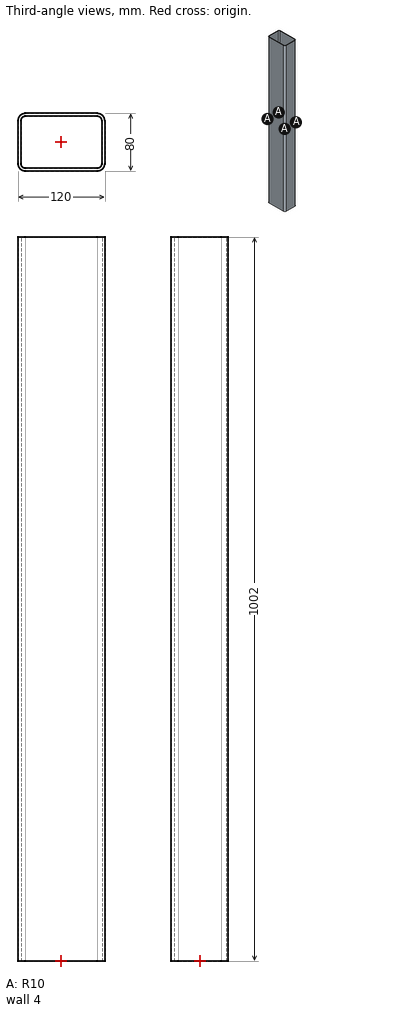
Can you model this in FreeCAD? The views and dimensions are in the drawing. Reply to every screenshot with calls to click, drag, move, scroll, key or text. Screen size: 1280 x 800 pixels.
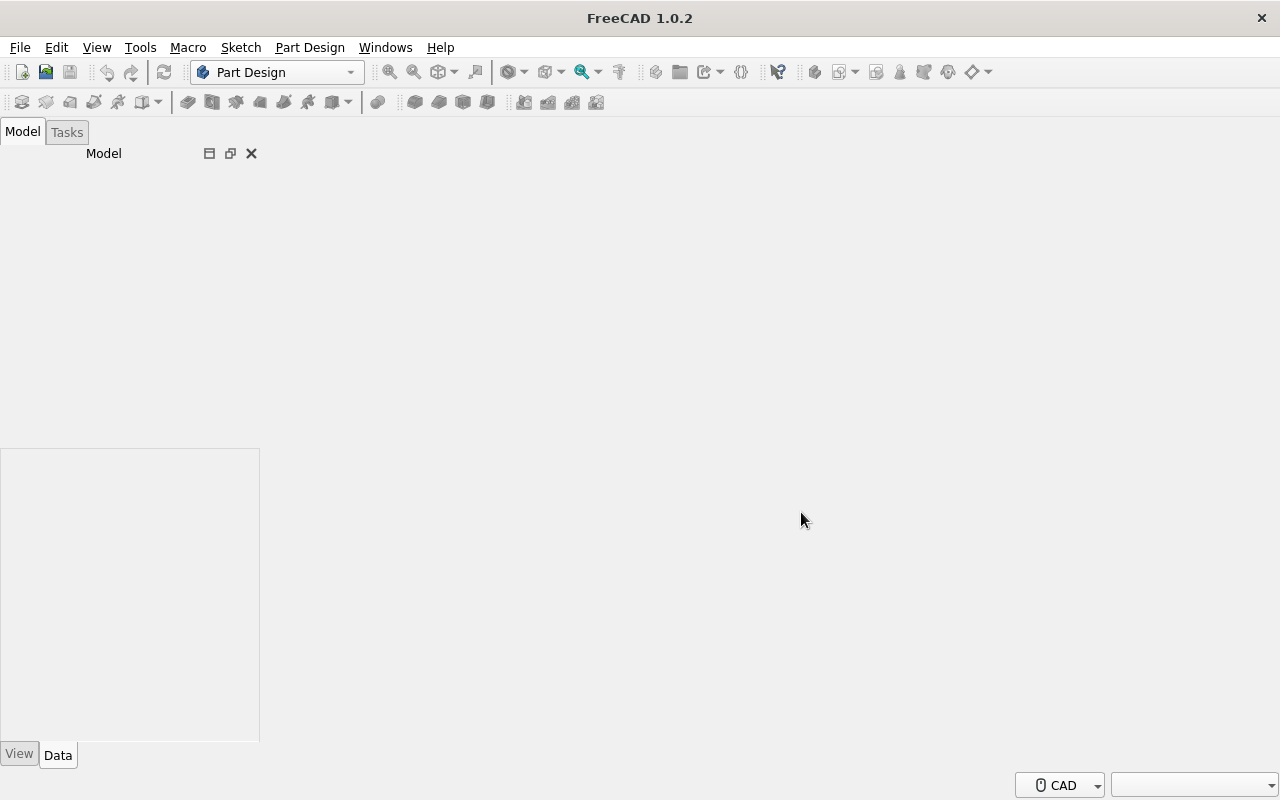
click(22, 72)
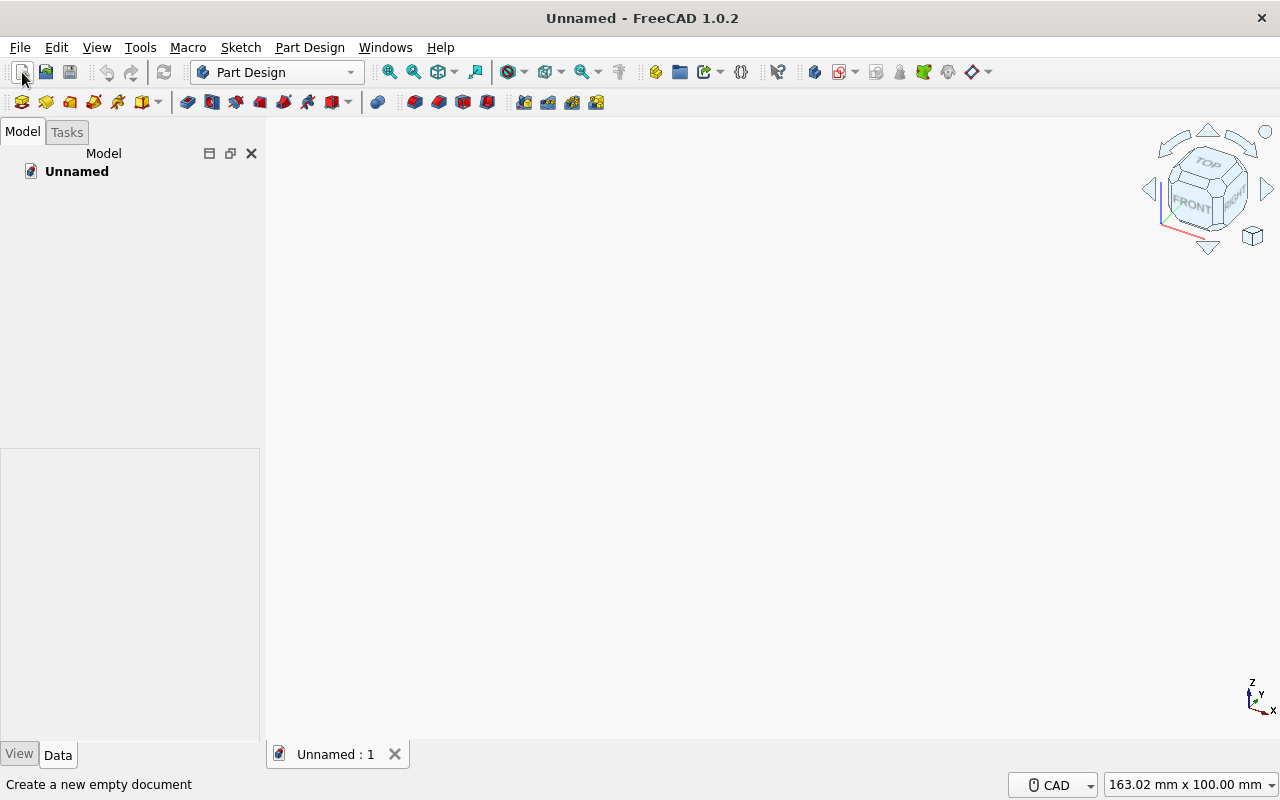
click(840, 72)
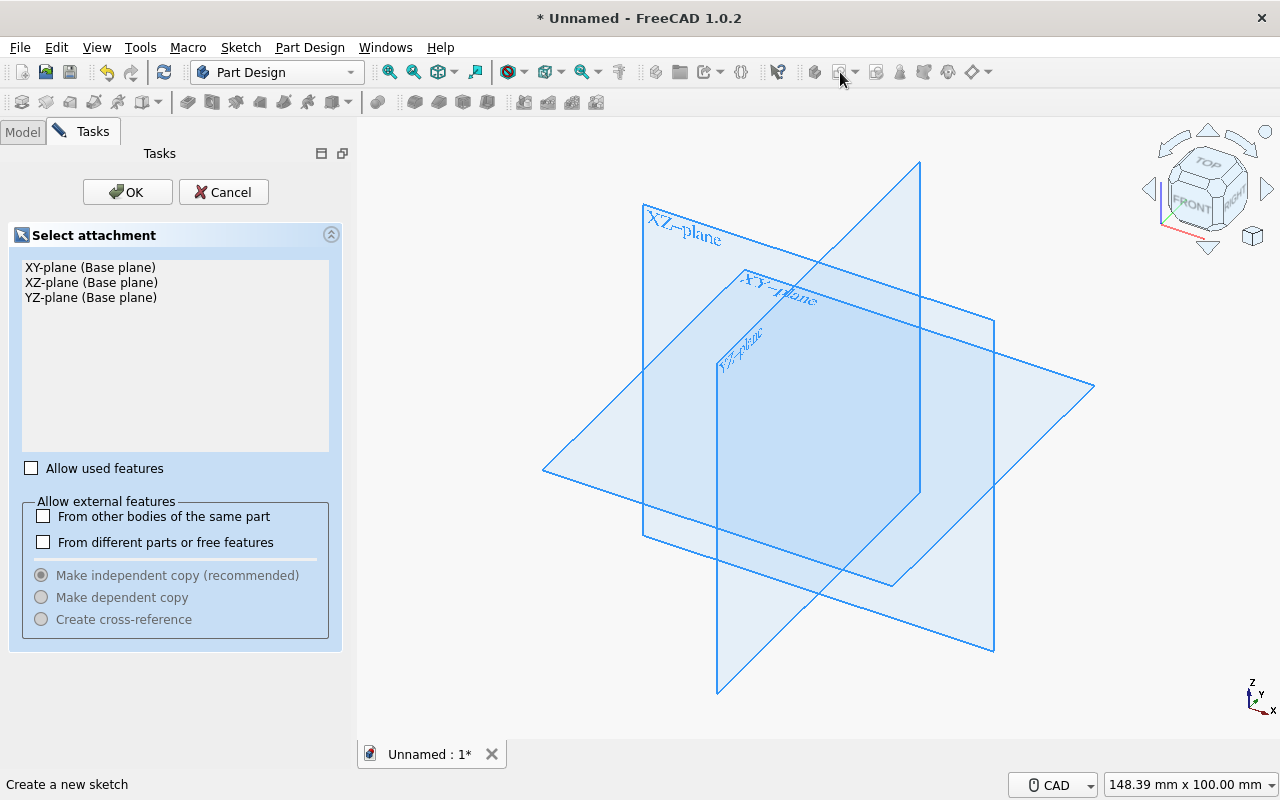
click(82, 268)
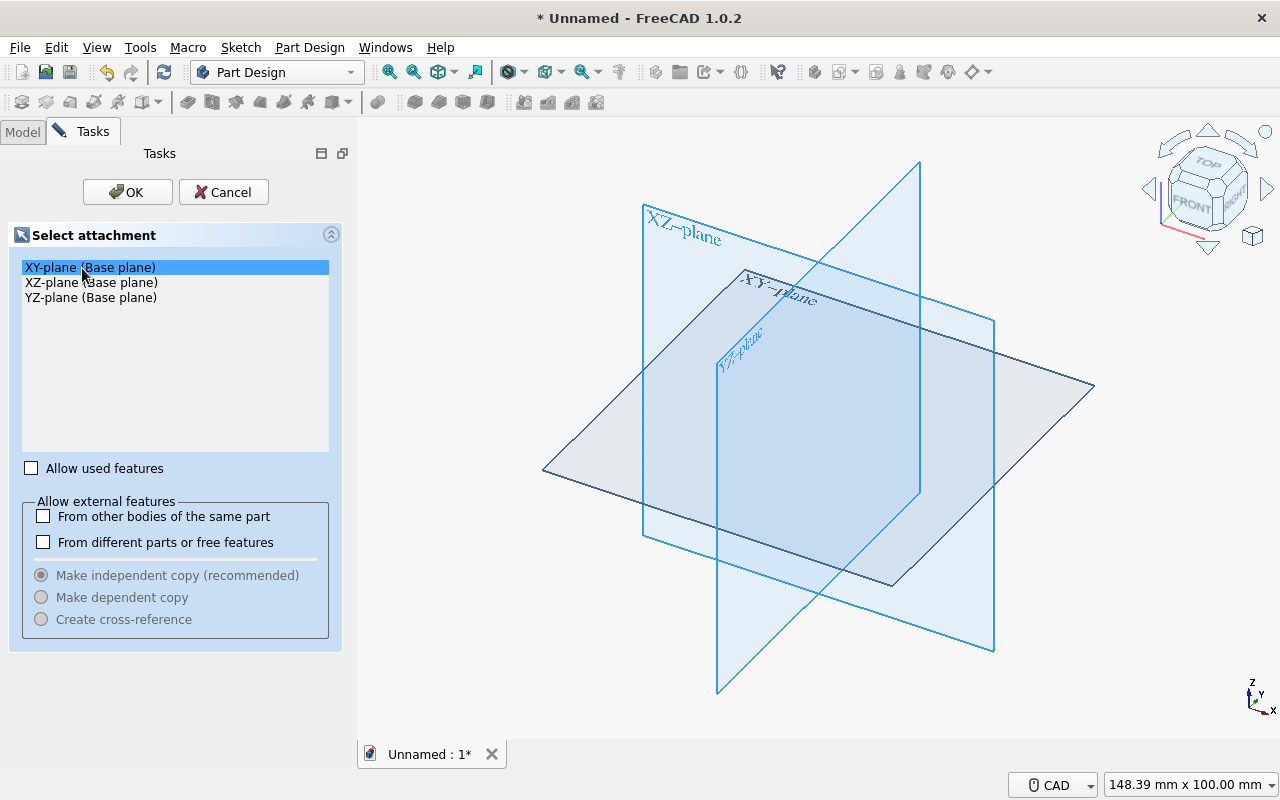
click(128, 192)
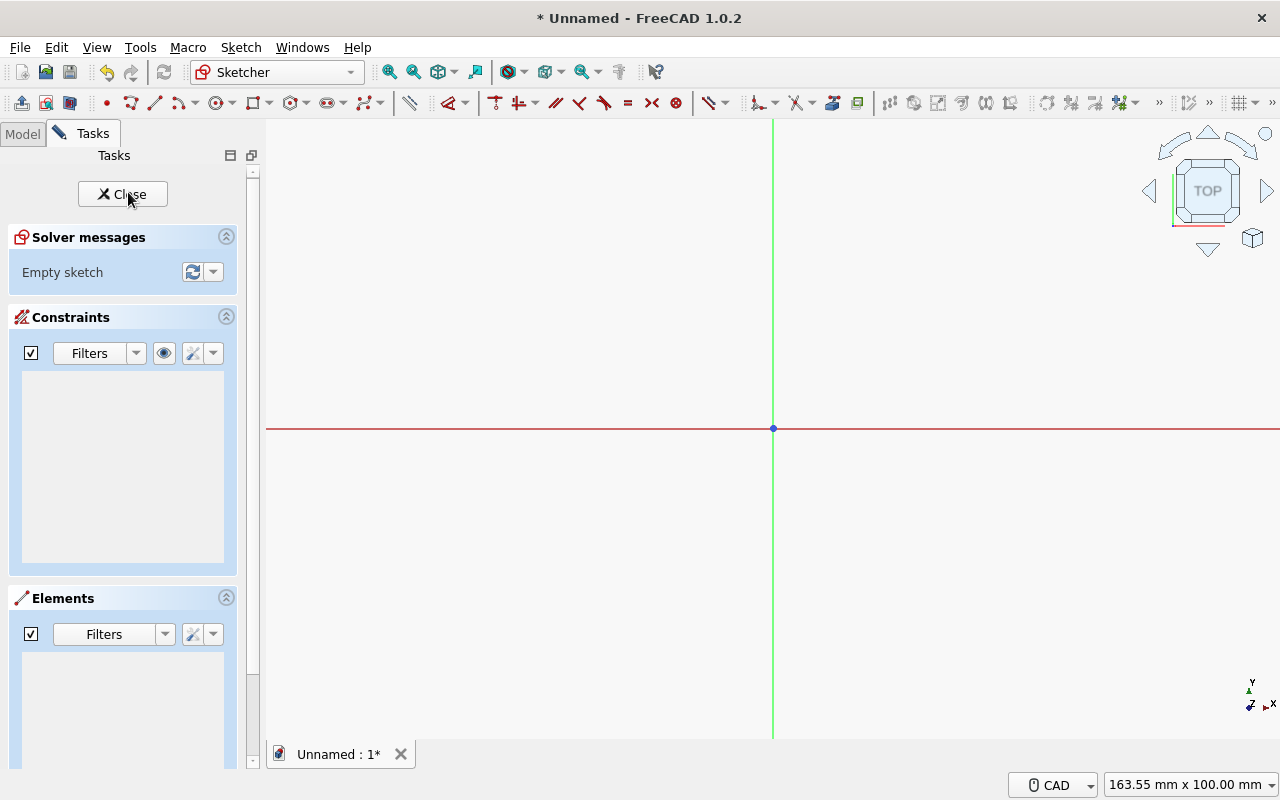
scroll(395, 429, down, 1)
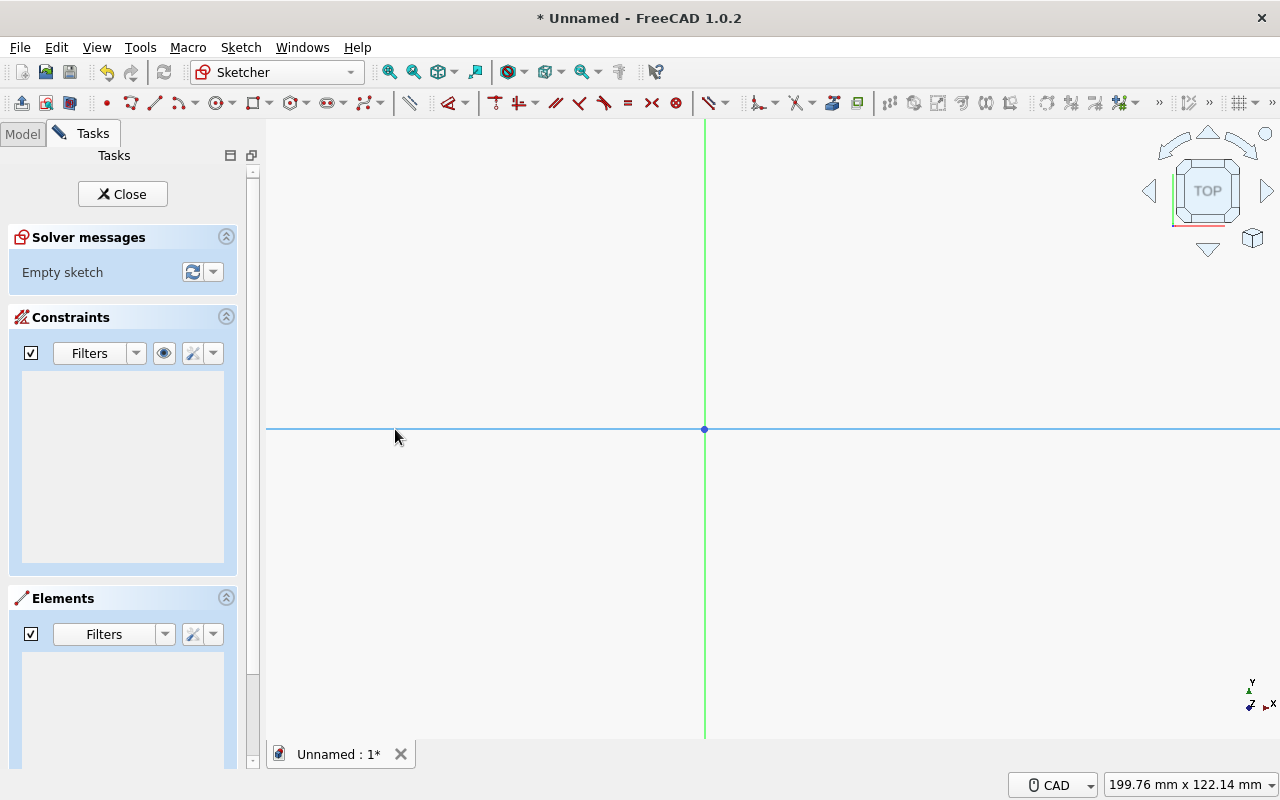
click(272, 104)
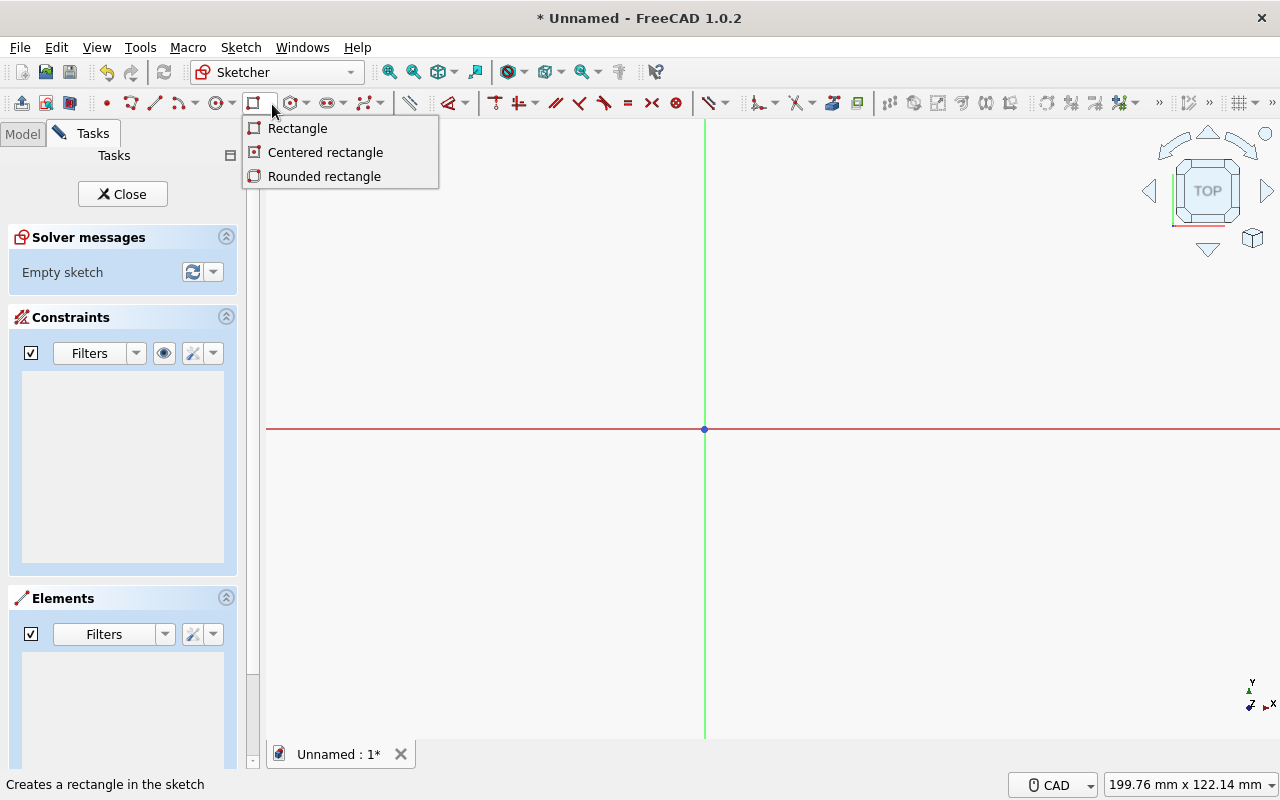
click(340, 152)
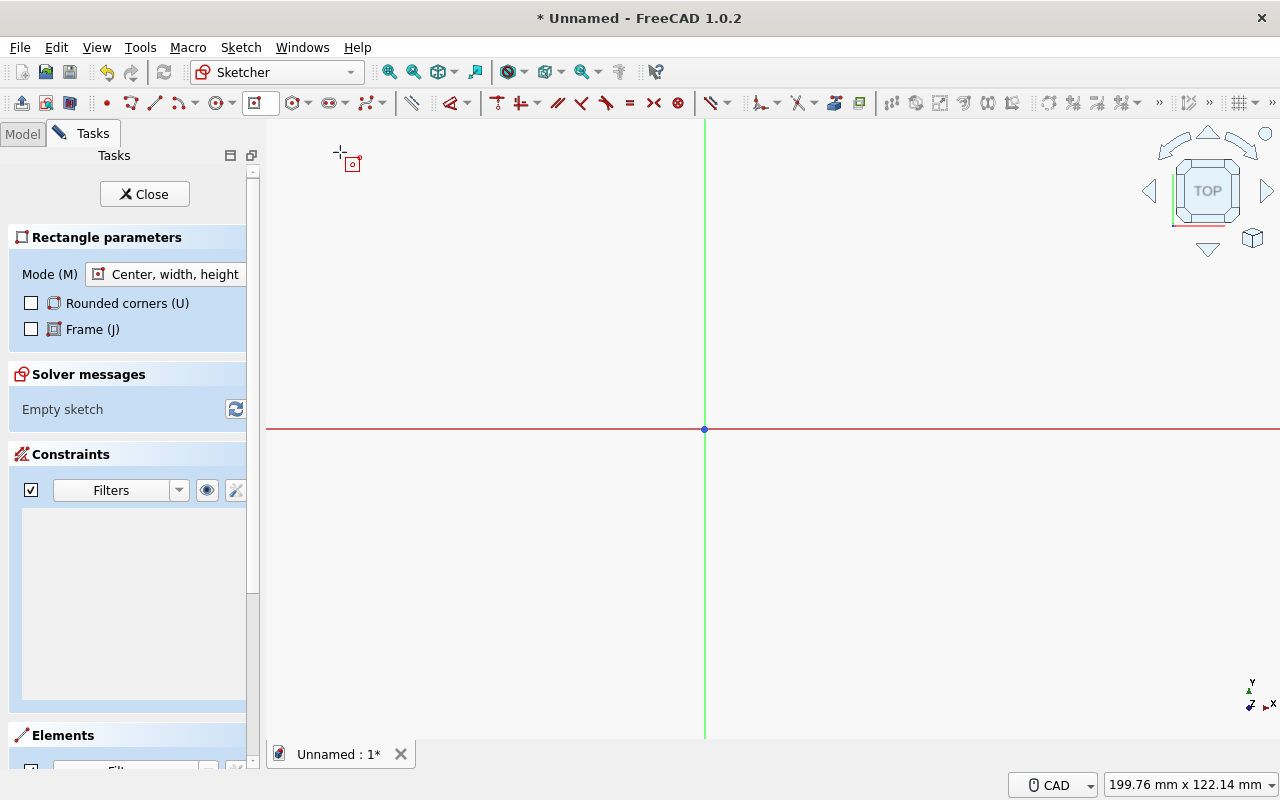
click(705, 429)
click(1009, 226)
key(Escape)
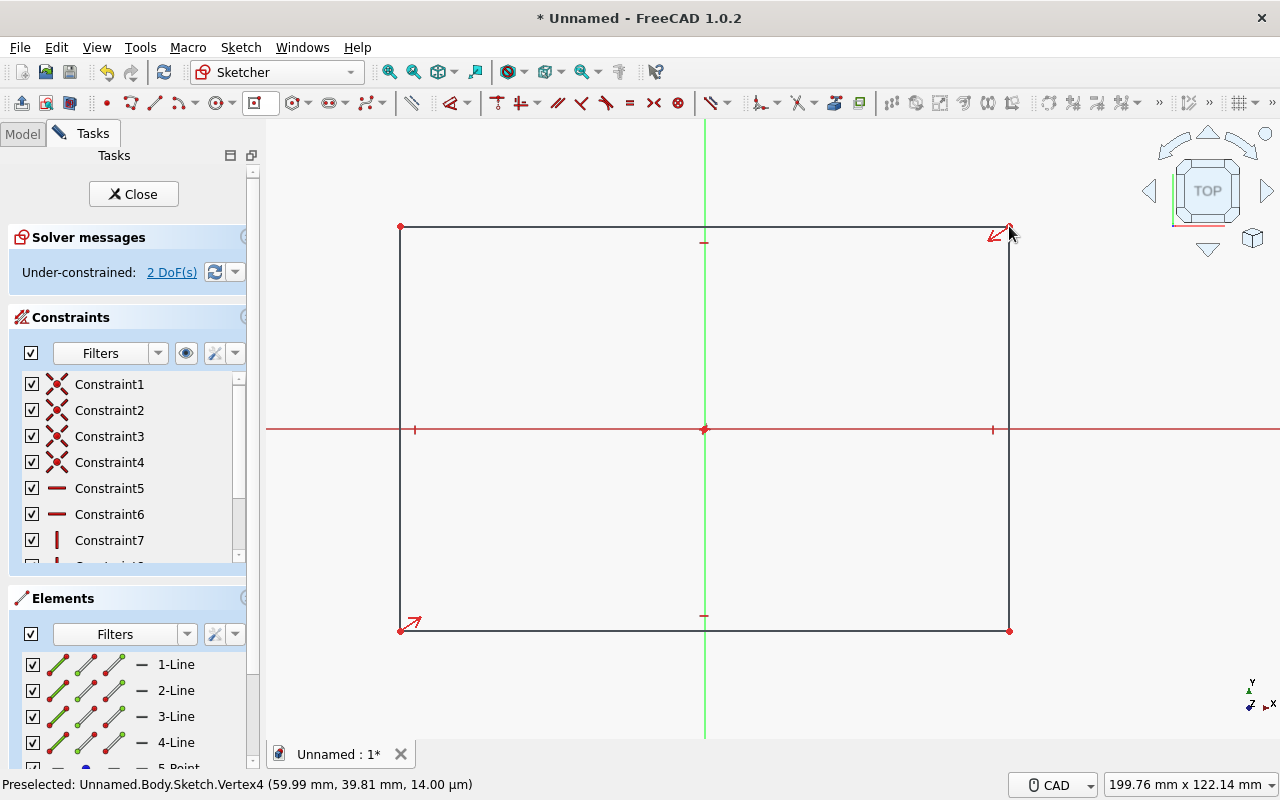
click(1009, 510)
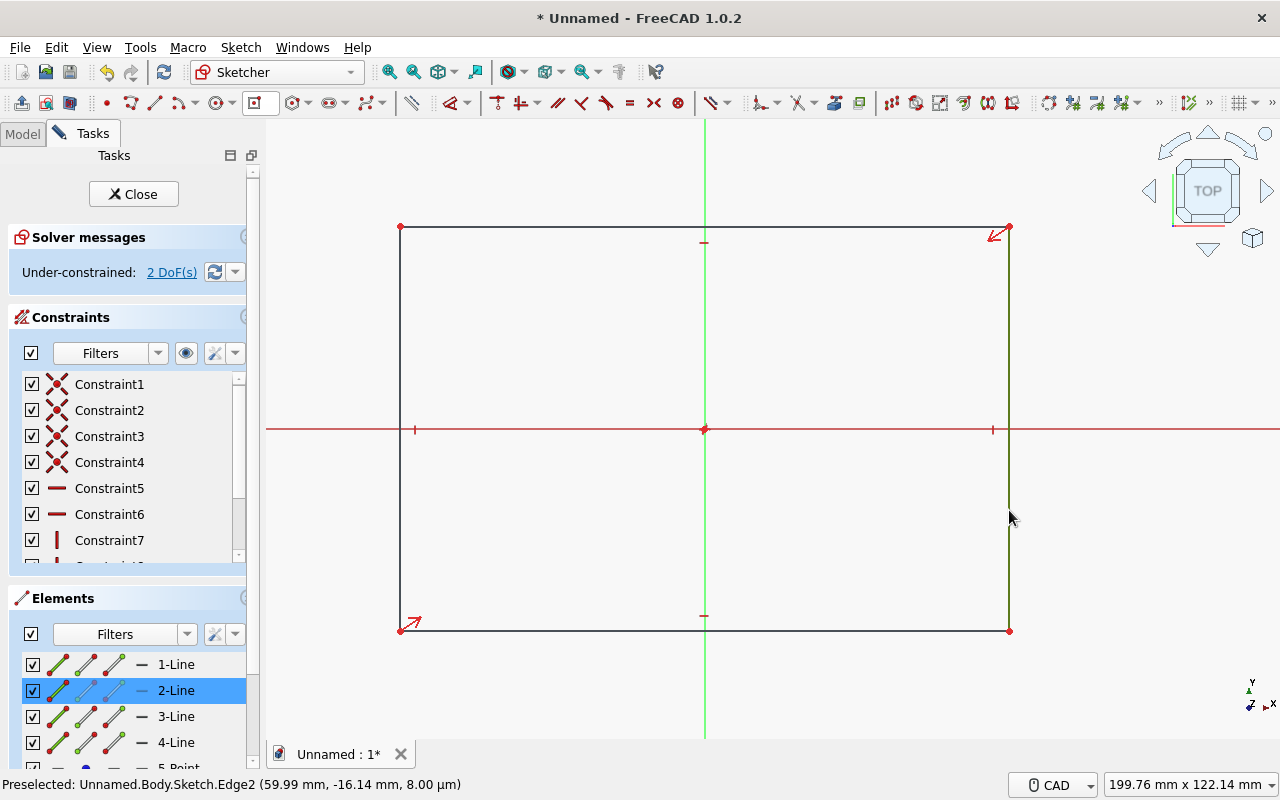
click(470, 104)